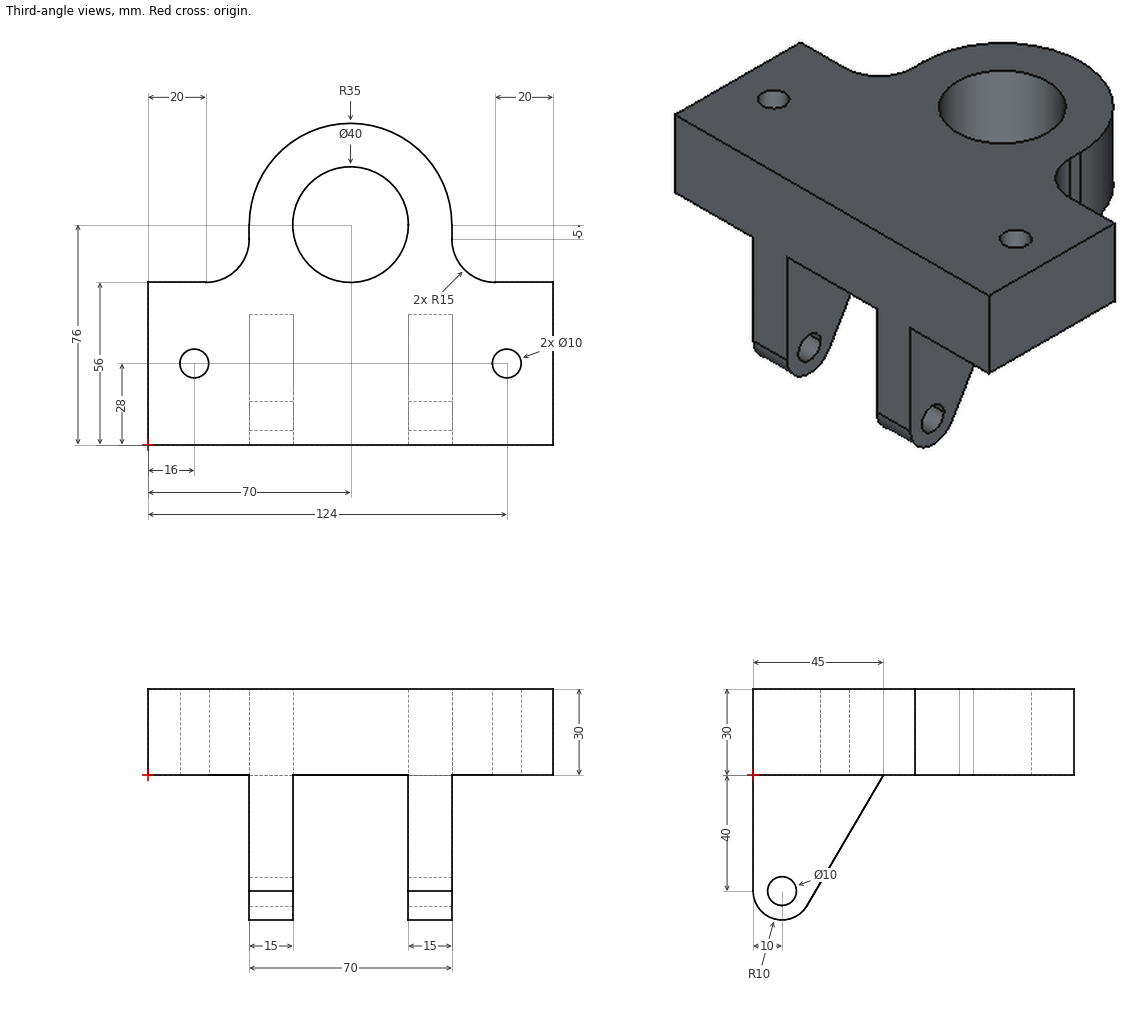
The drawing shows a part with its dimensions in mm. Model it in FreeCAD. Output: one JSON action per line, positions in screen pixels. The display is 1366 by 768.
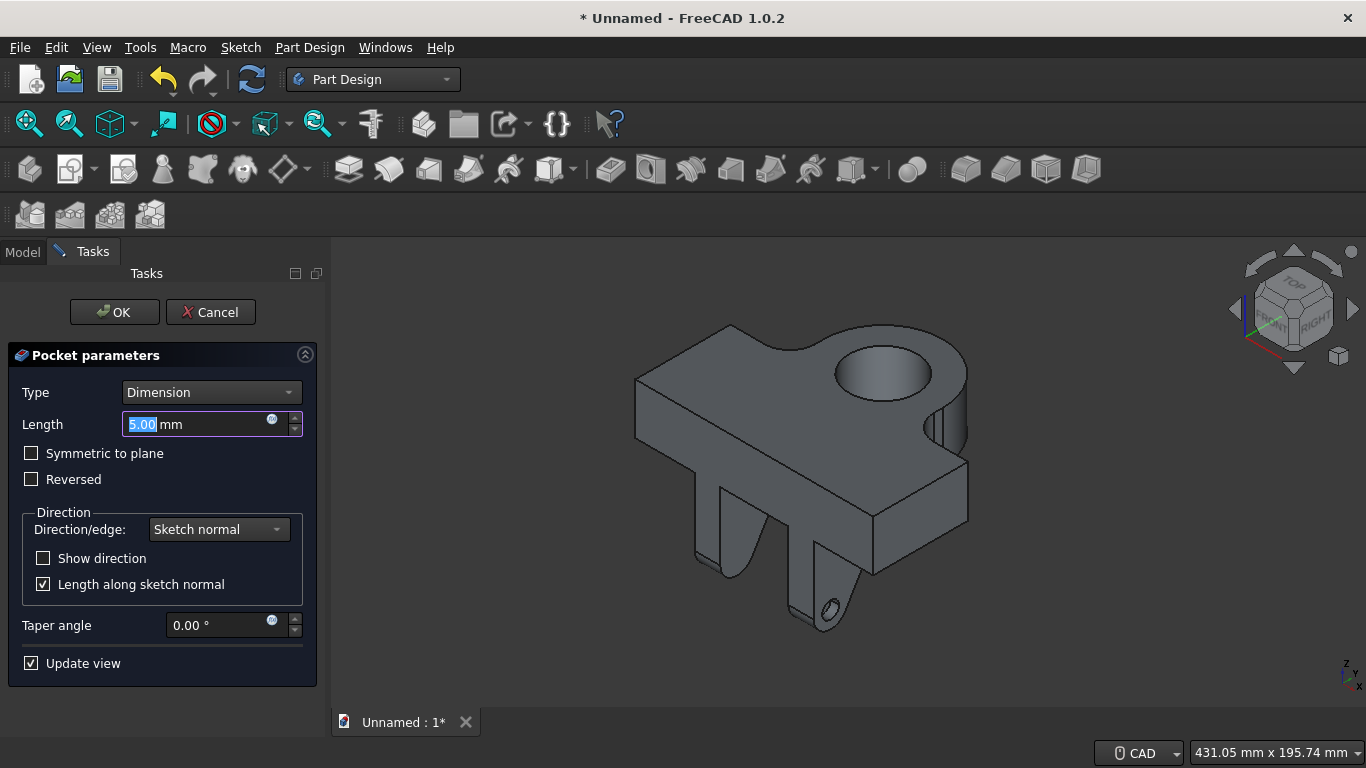
{"action": "type", "text": "70"}
{"action": "key", "text": "Tab"}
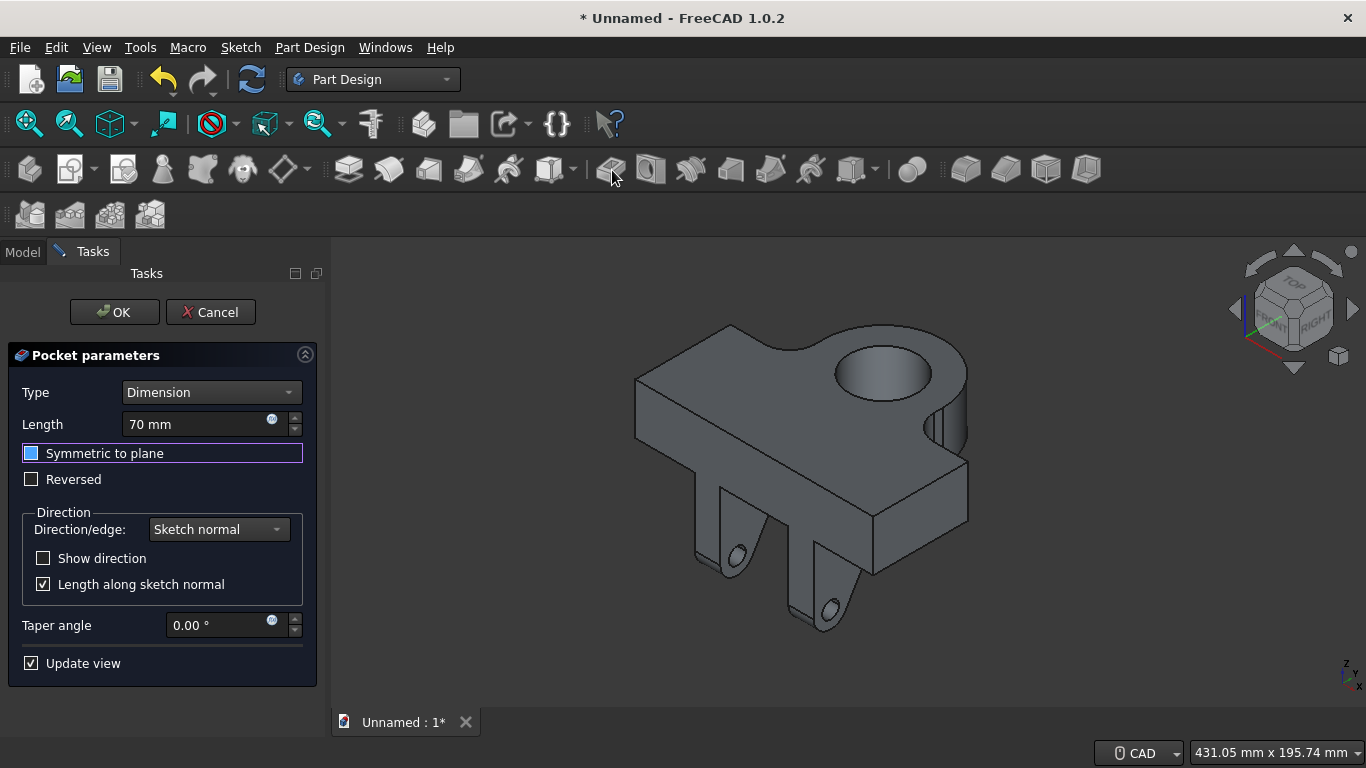
{"action": "left_click", "coordinate": [115, 312]}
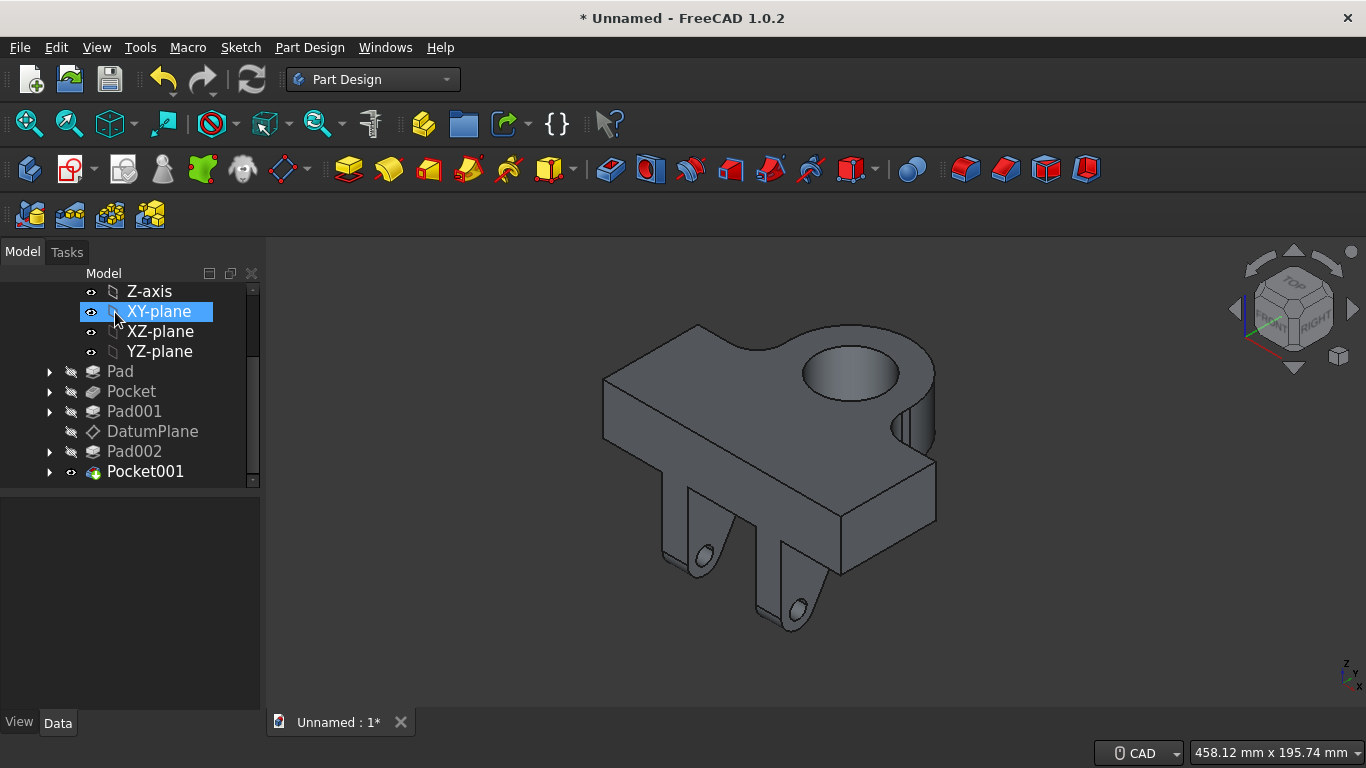
{"action": "key", "text": "5"}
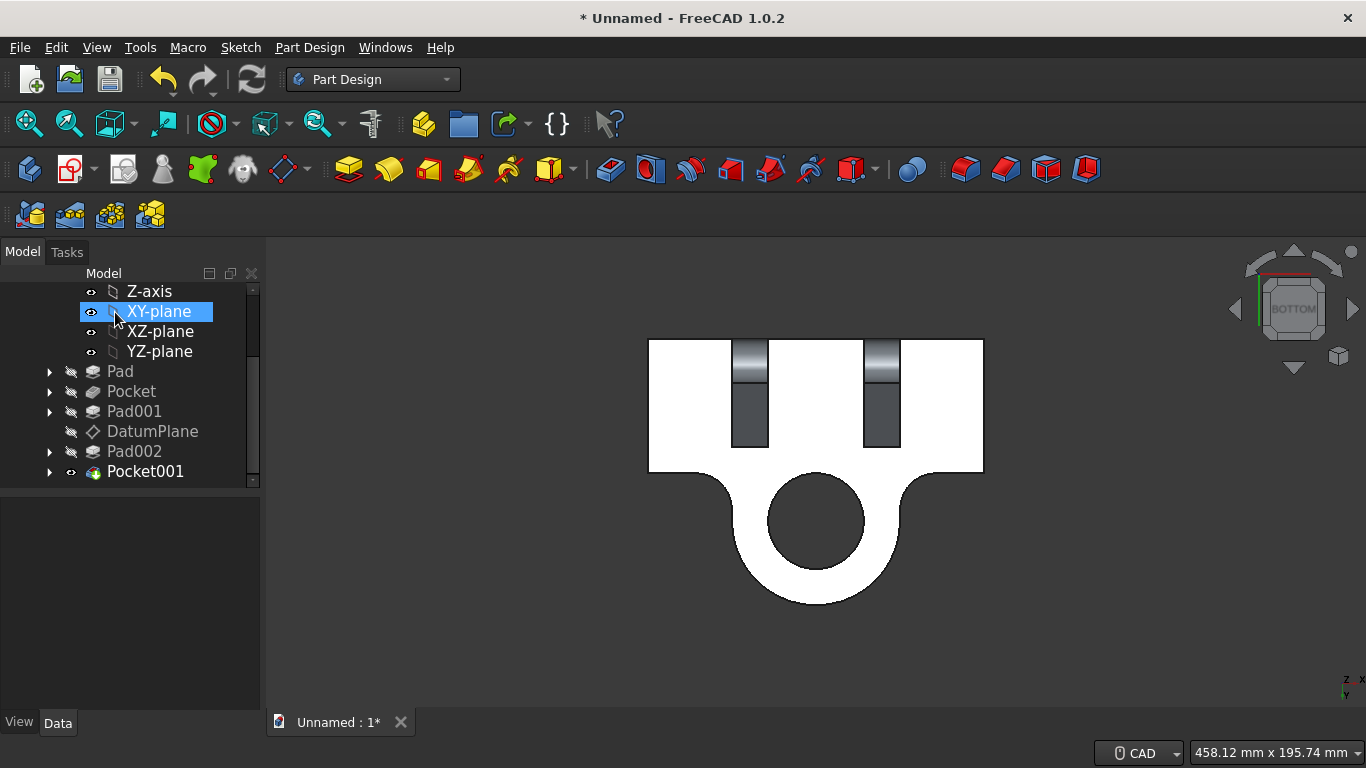
{"action": "left_click", "coordinate": [816, 395]}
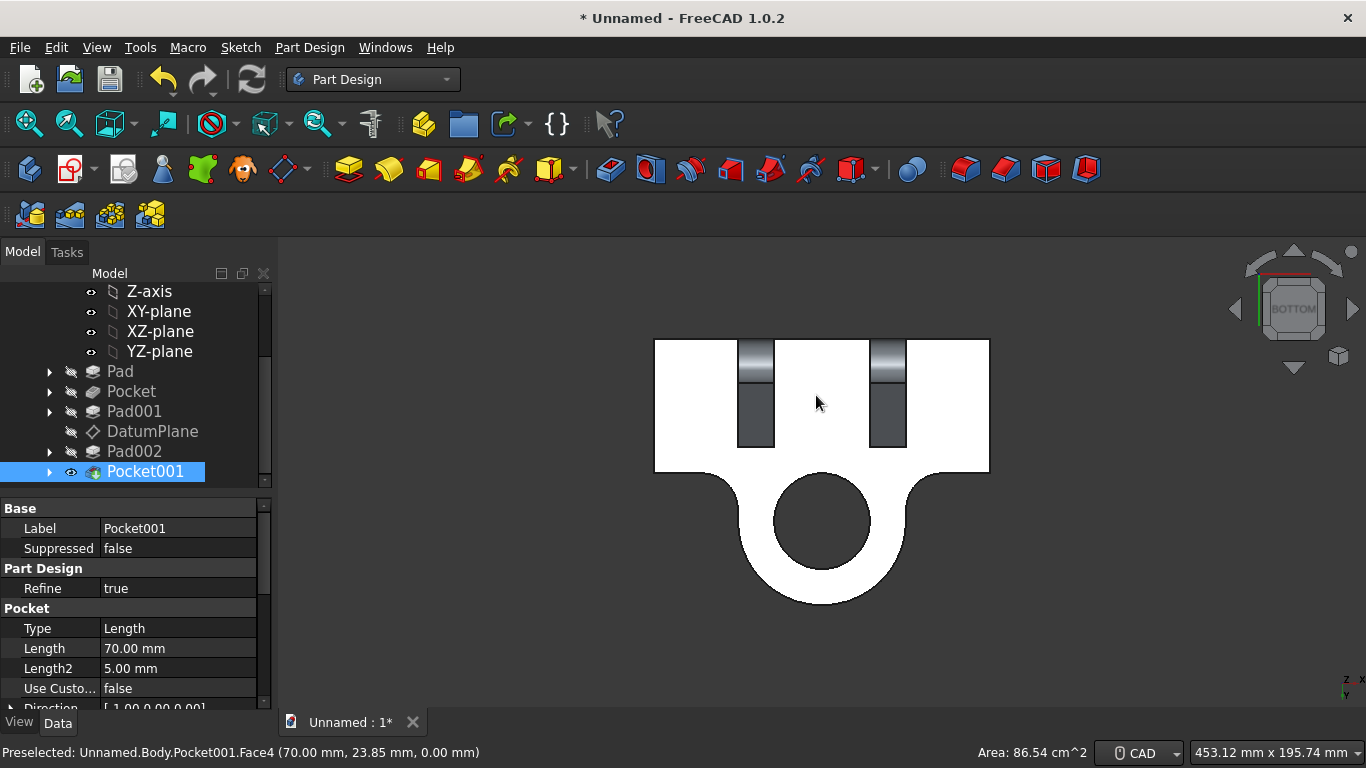
{"action": "left_click", "coordinate": [70, 170]}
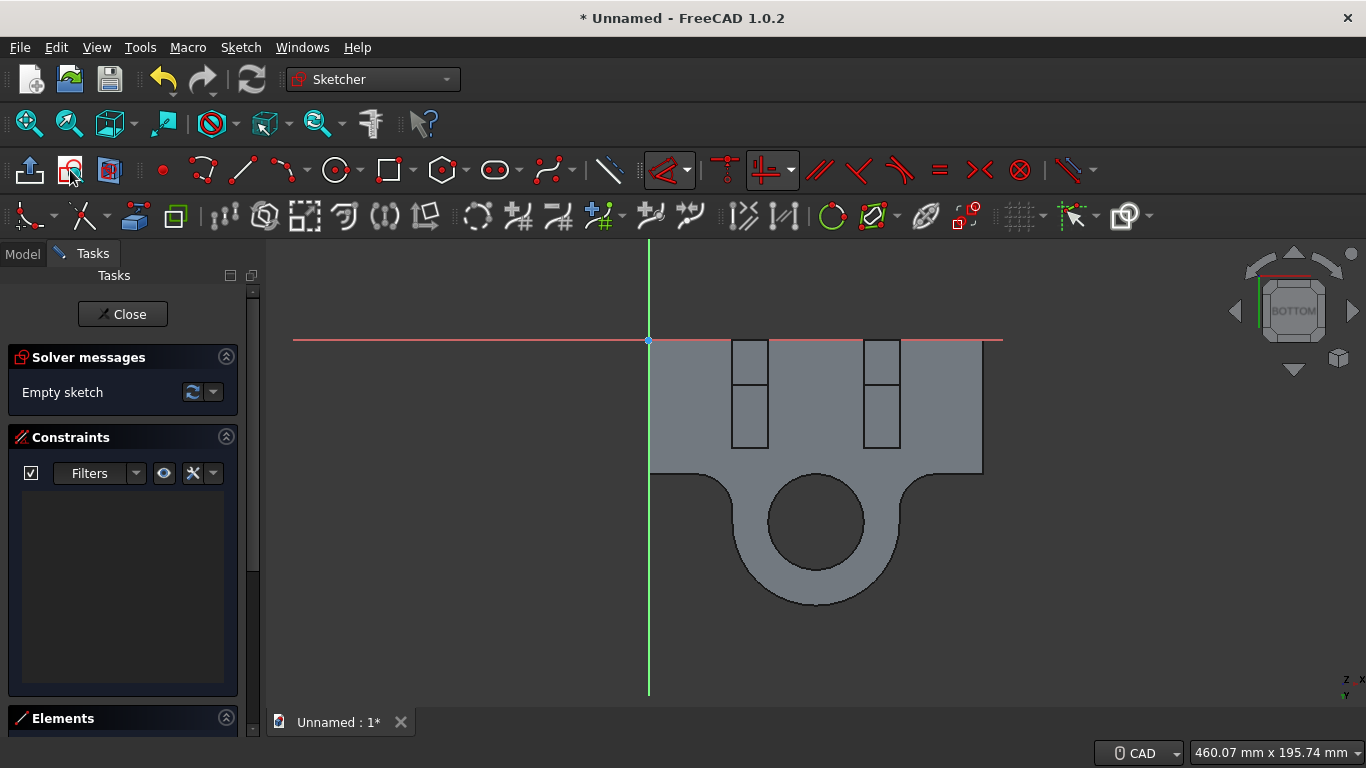
{"action": "left_click", "coordinate": [110, 170]}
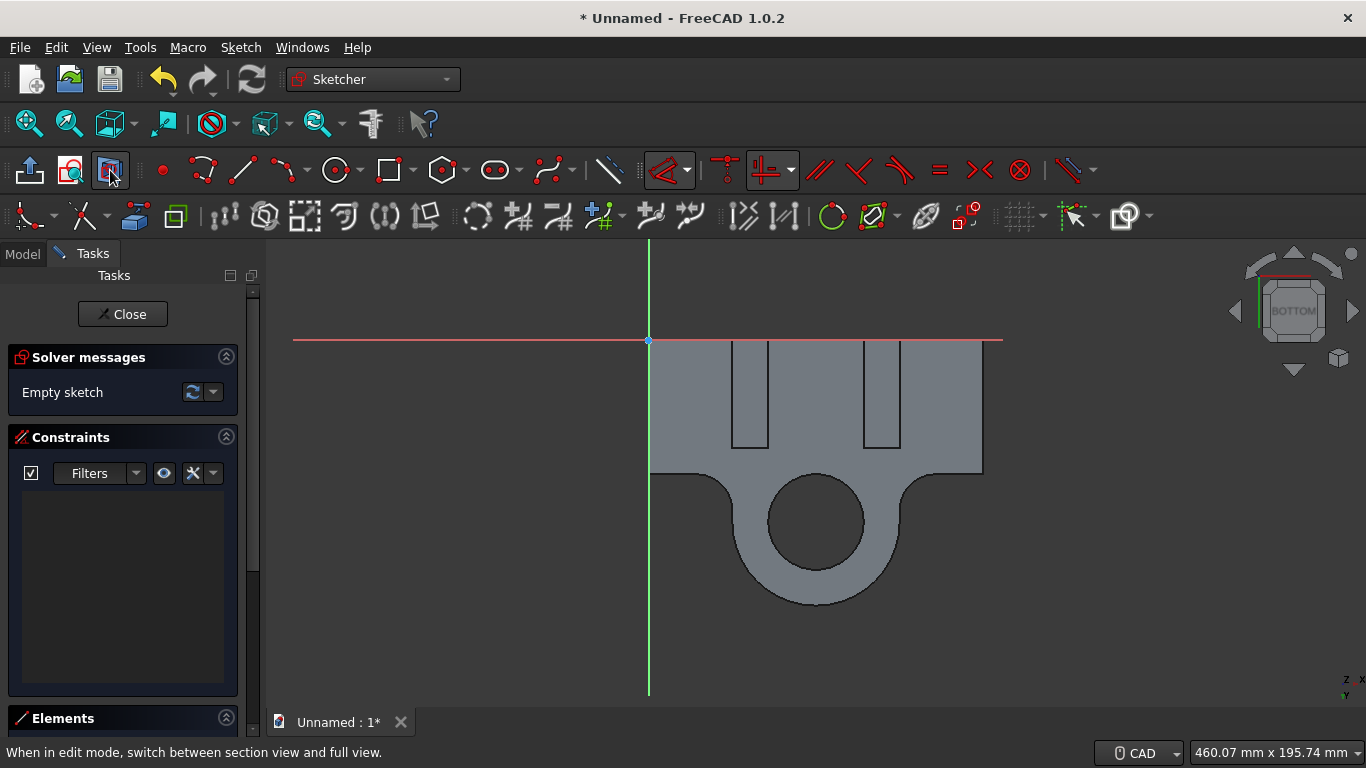
{"action": "scroll", "coordinate": [848, 304], "scroll_direction": "up", "scroll_amount": 4}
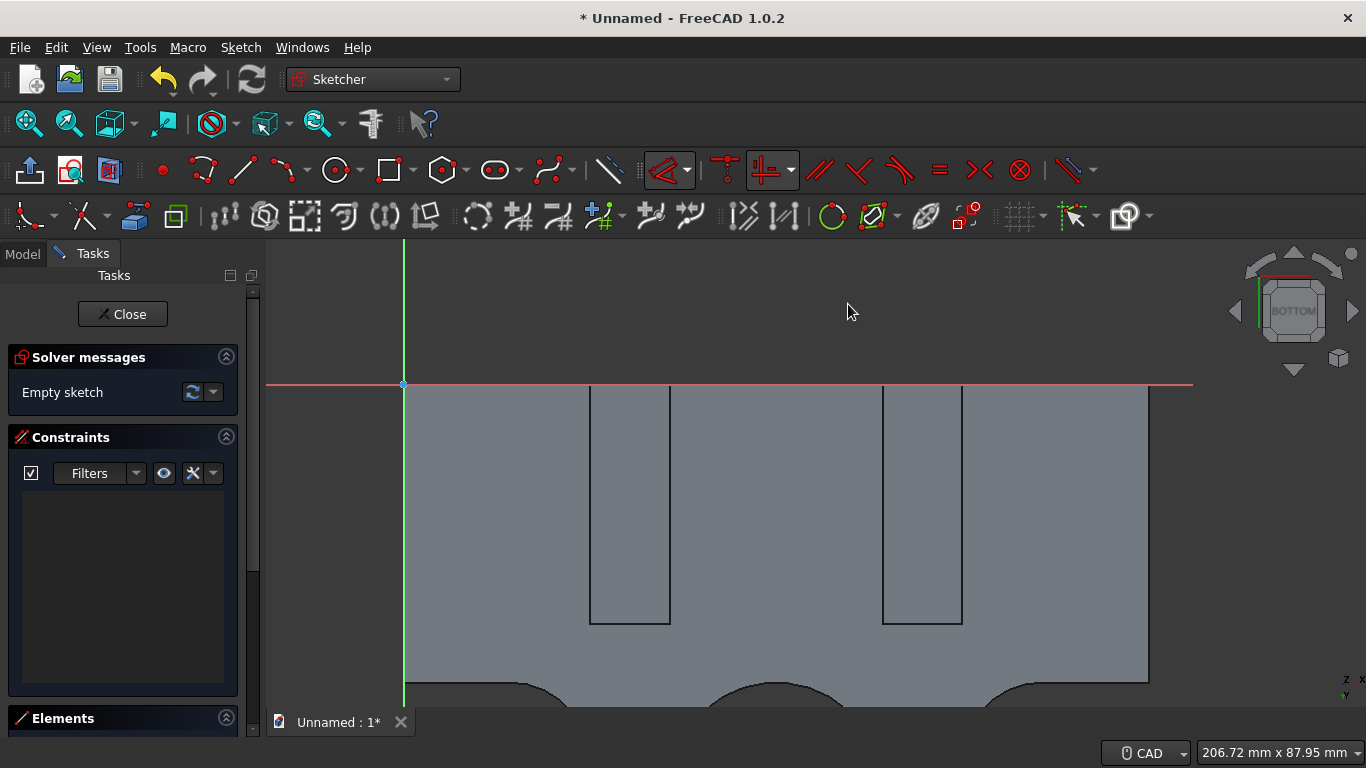
{"action": "left_click", "coordinate": [336, 170]}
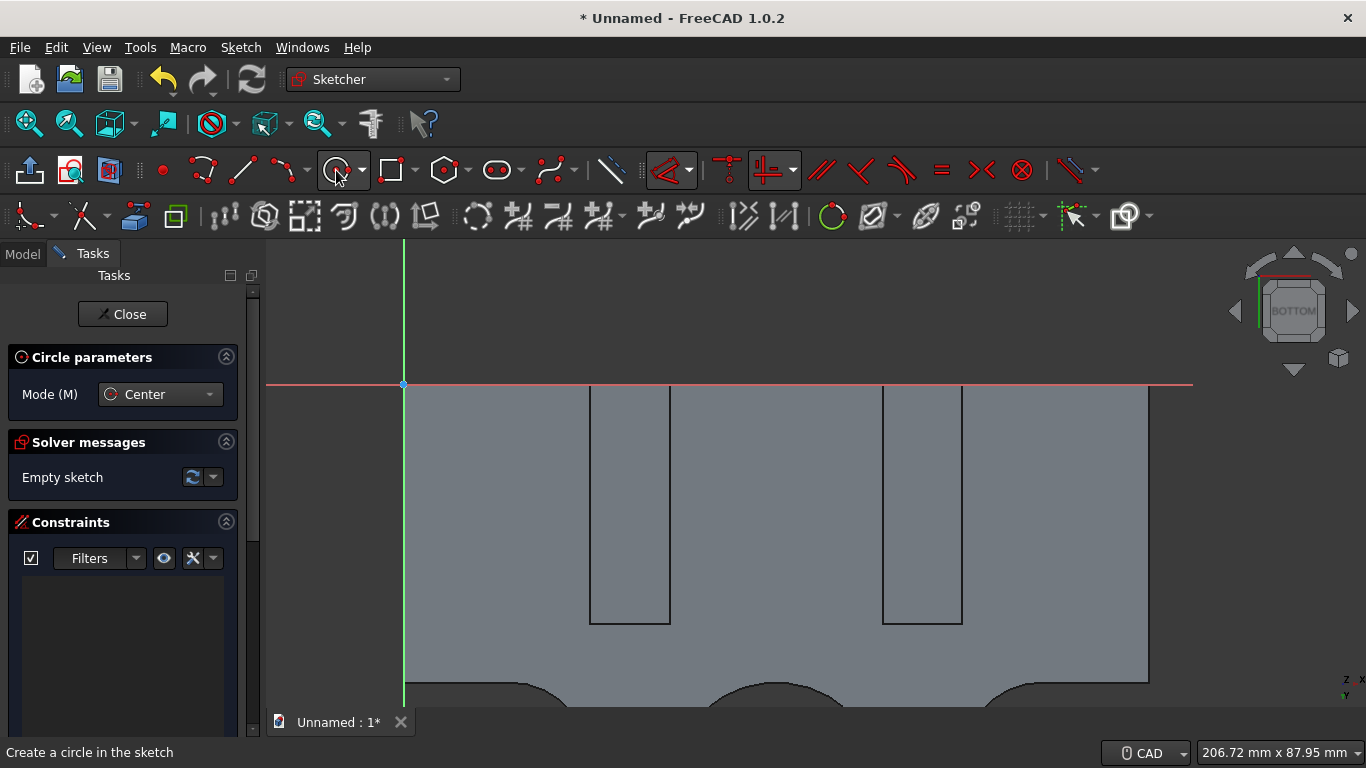
{"action": "left_click", "coordinate": [1063, 534]}
{"action": "mouse_move", "coordinate": [1082, 515]}